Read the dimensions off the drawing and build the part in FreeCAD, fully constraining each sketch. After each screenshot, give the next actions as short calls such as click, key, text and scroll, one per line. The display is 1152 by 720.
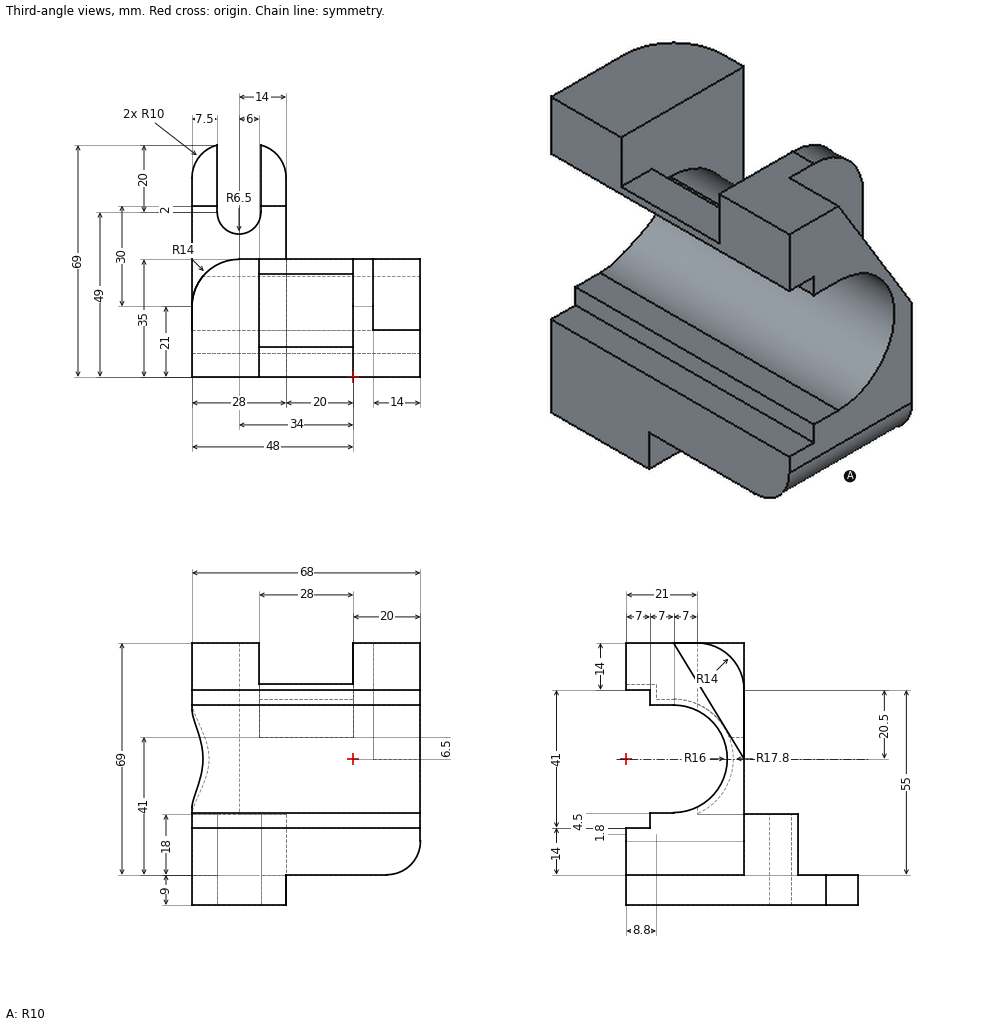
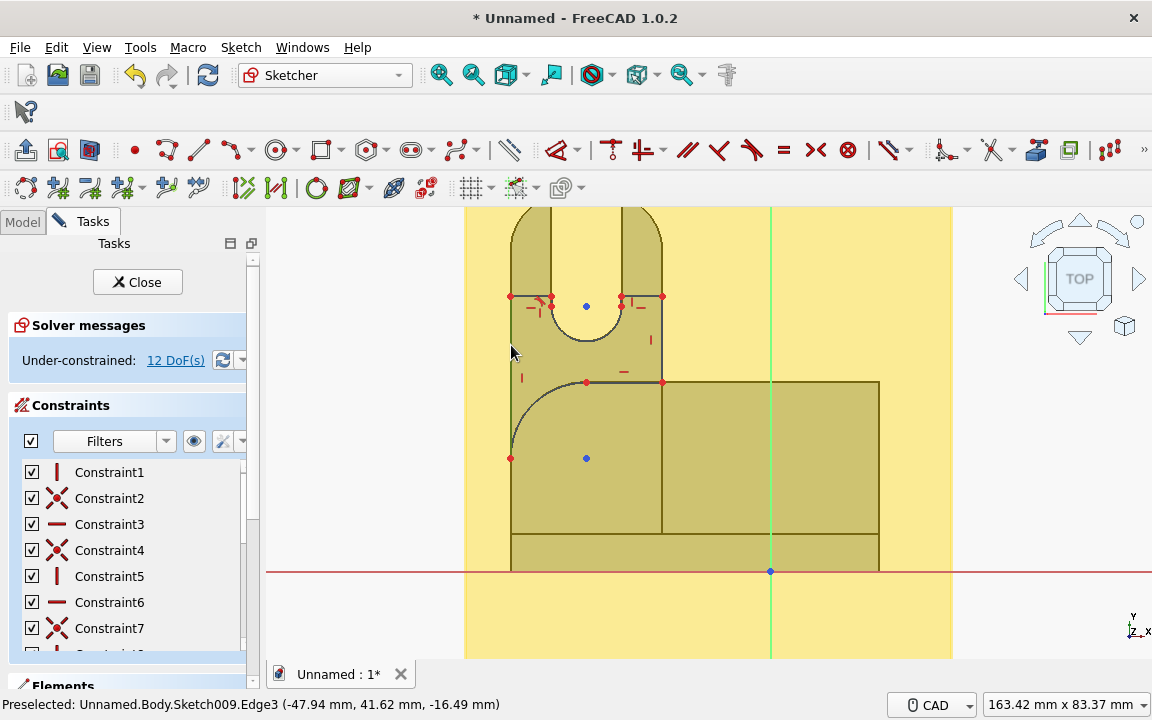
click(552, 391)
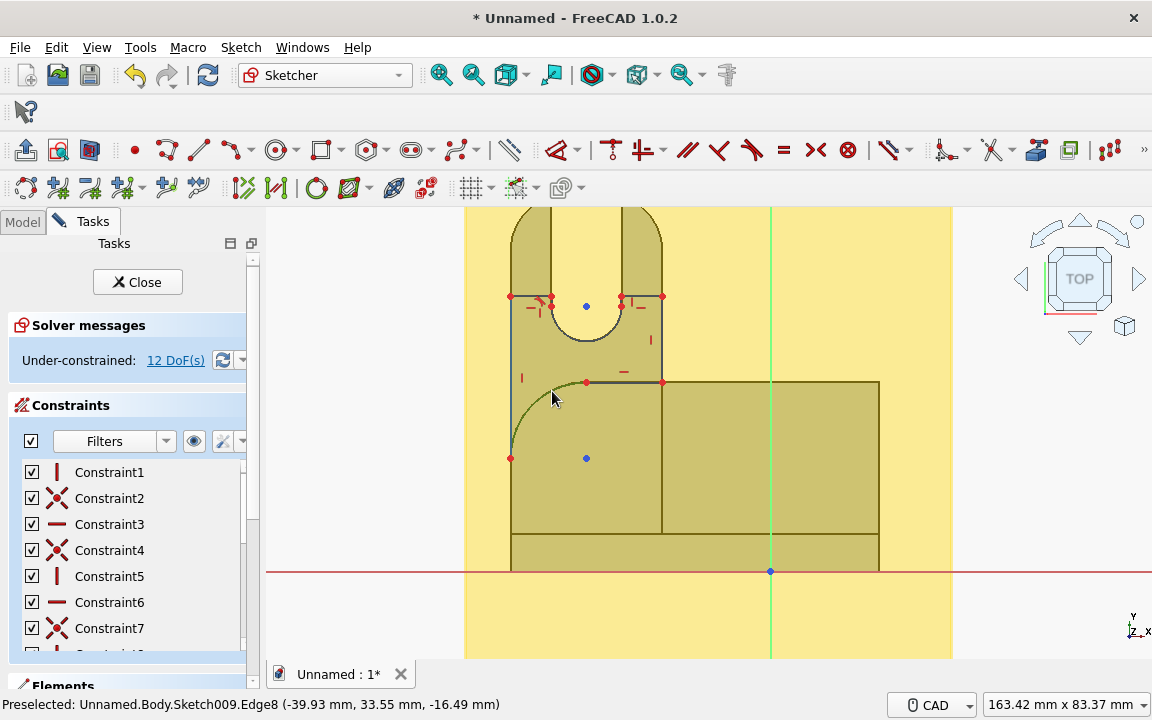
click(752, 150)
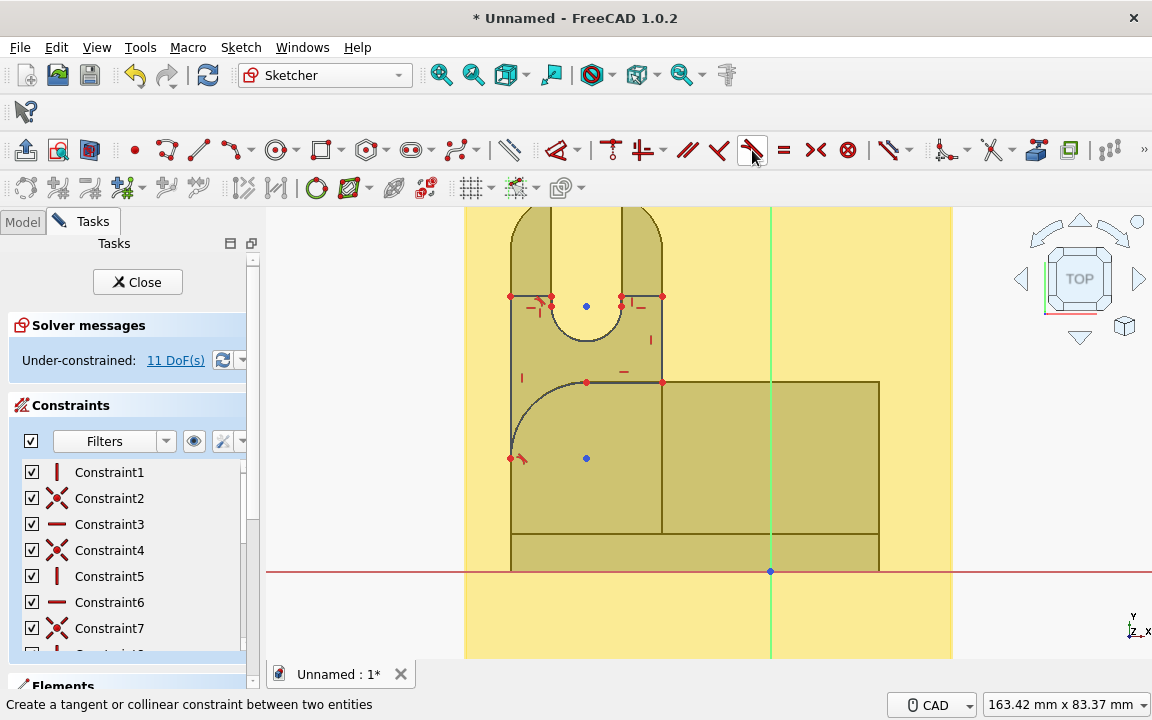
click(609, 383)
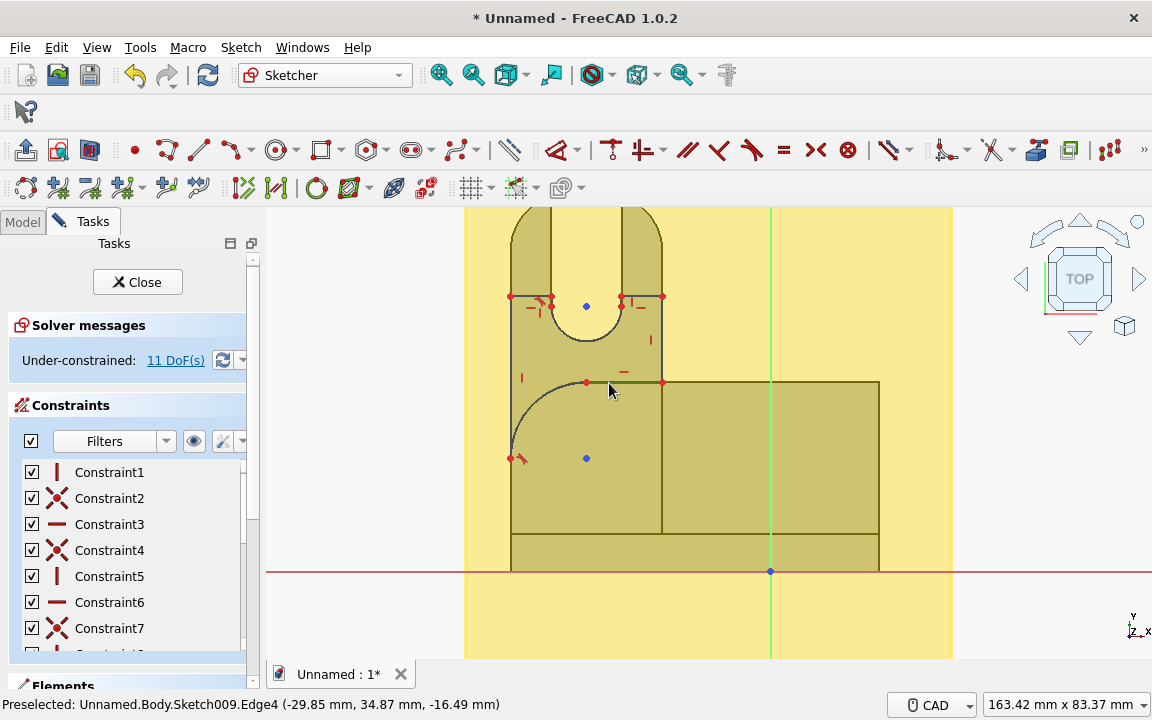
click(552, 391)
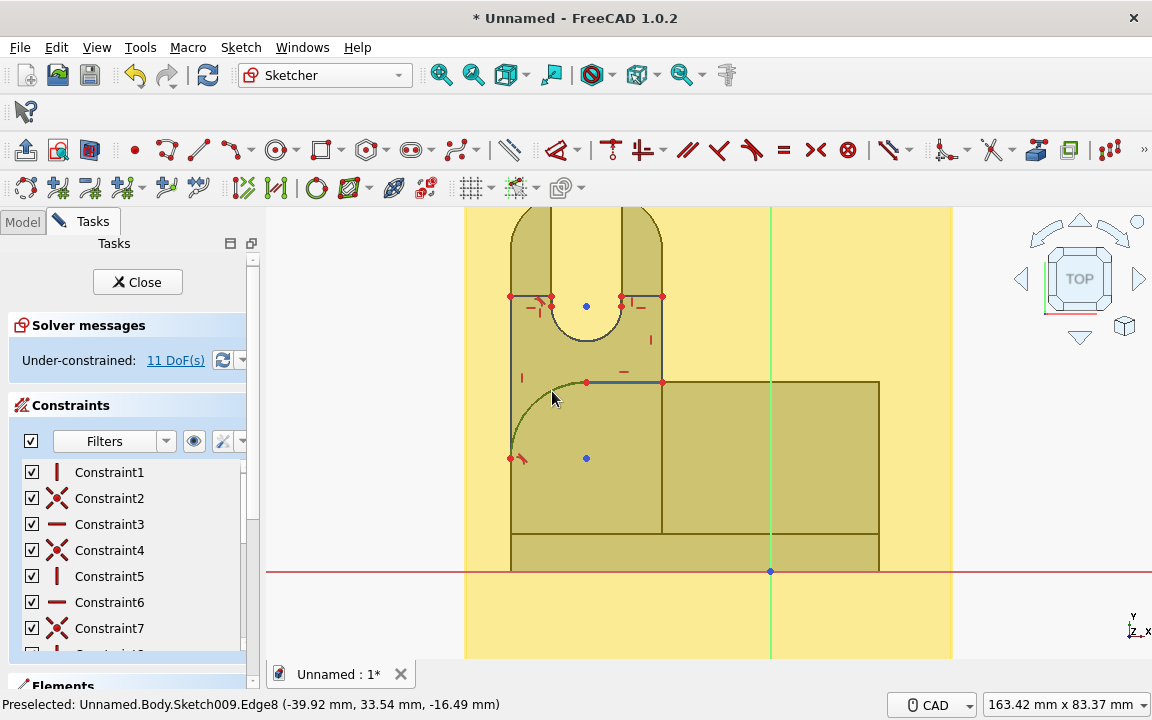
key(t)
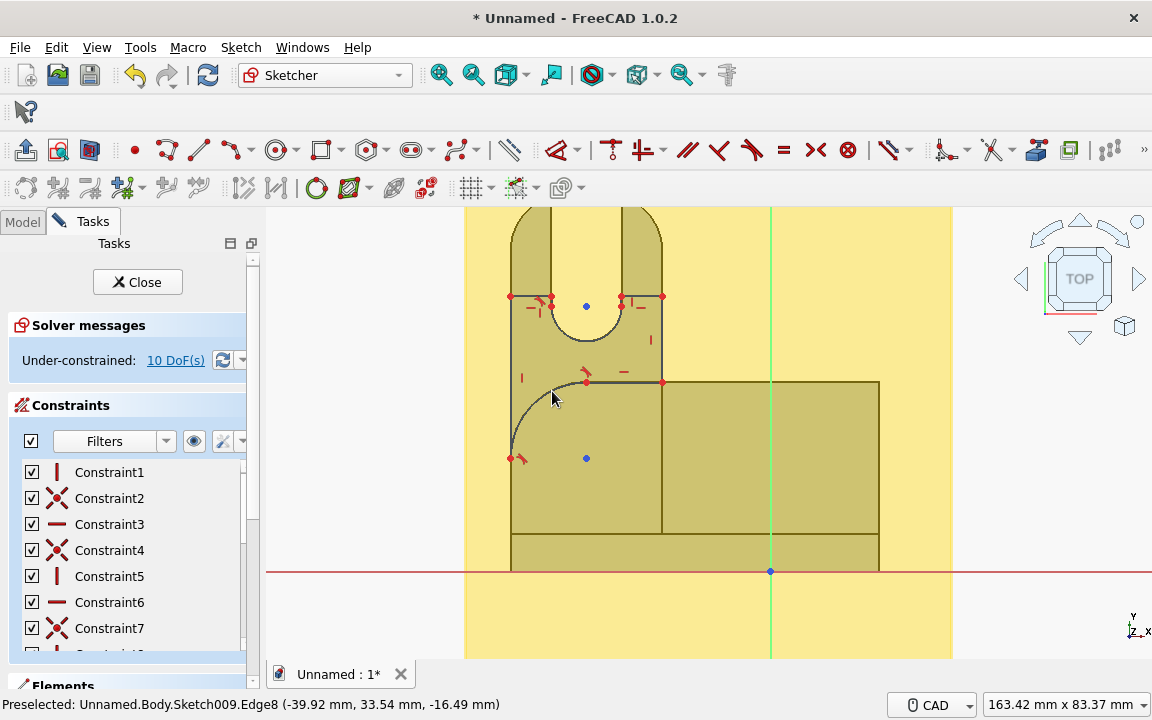
scroll(621, 301, up, 5)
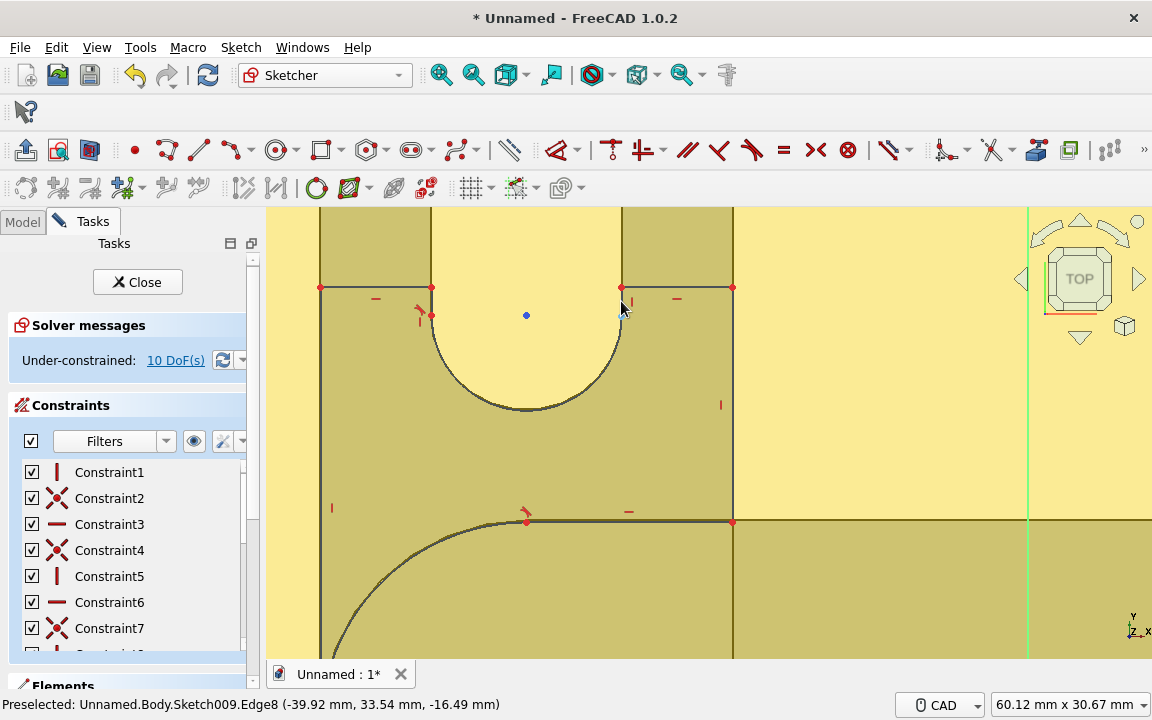
click(622, 302)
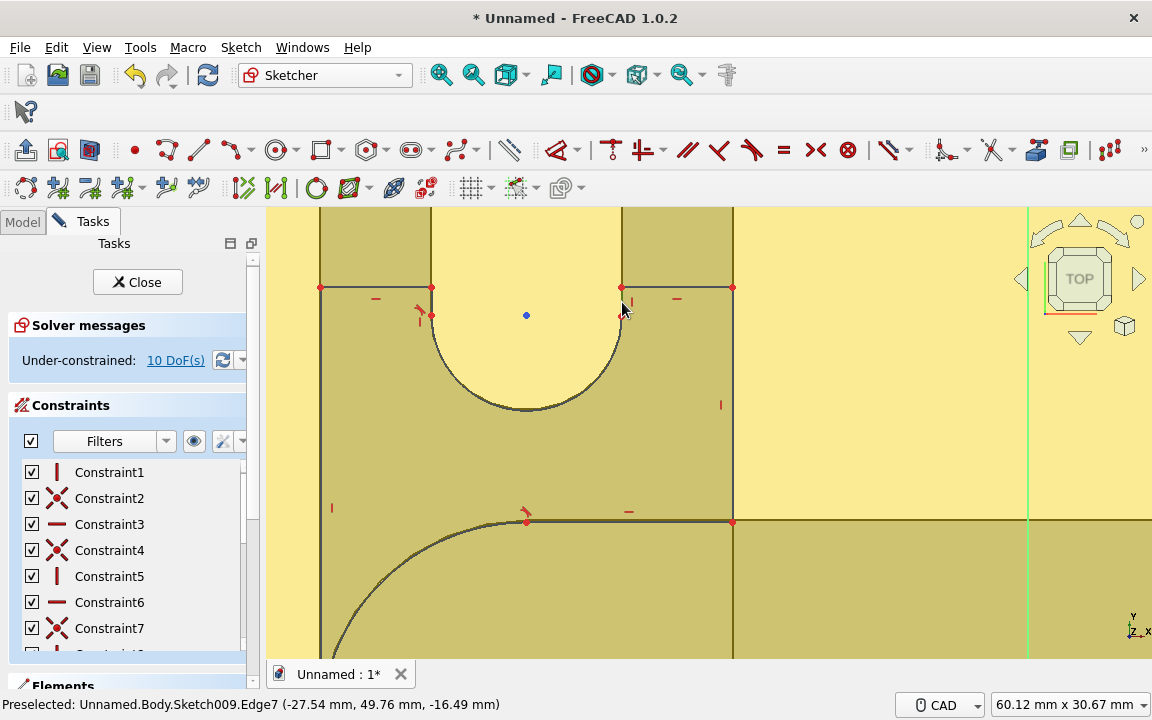
click(471, 392)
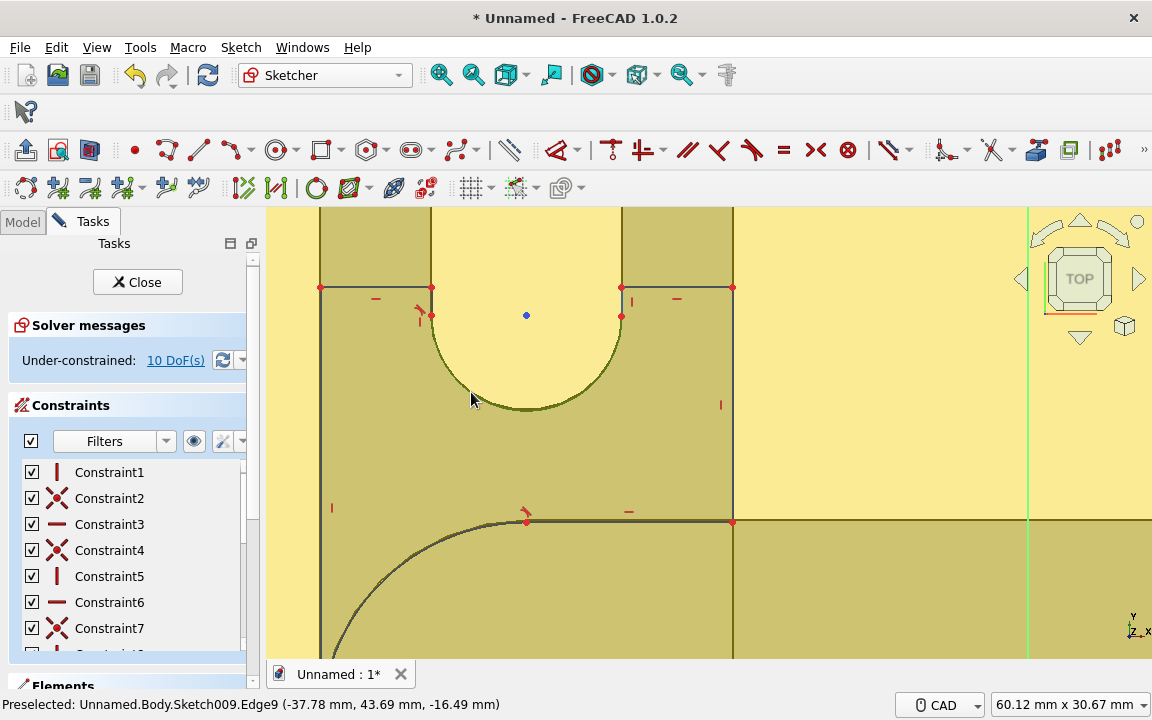
click(752, 150)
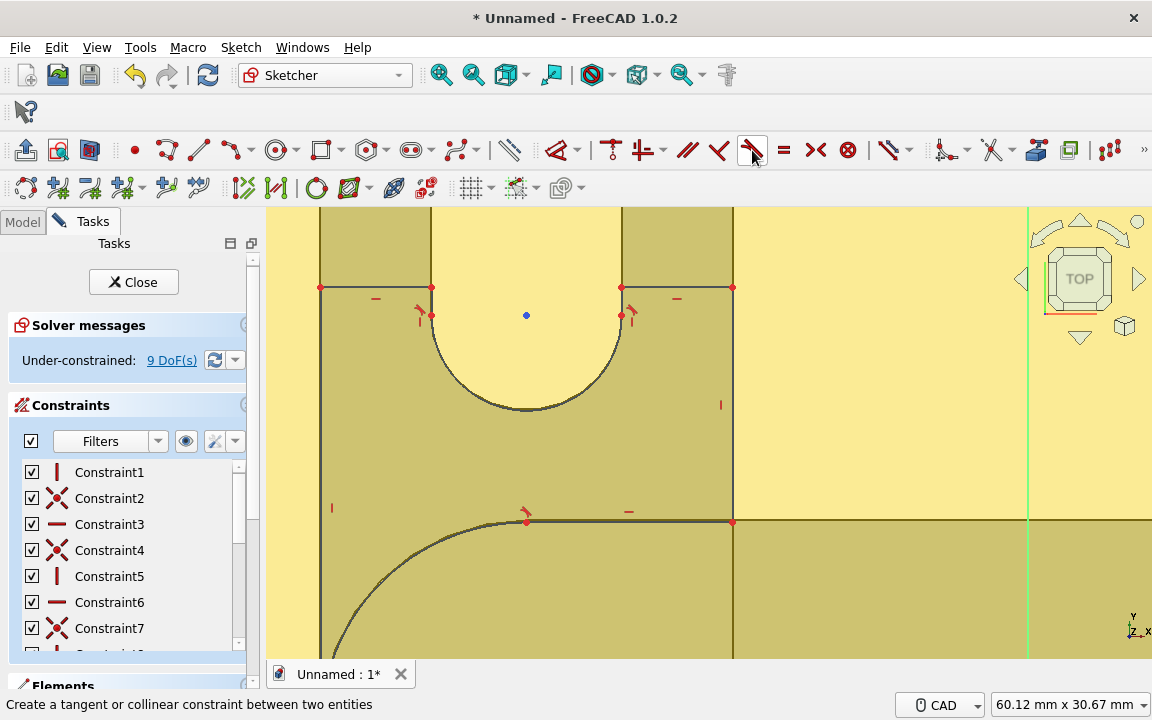
click(556, 150)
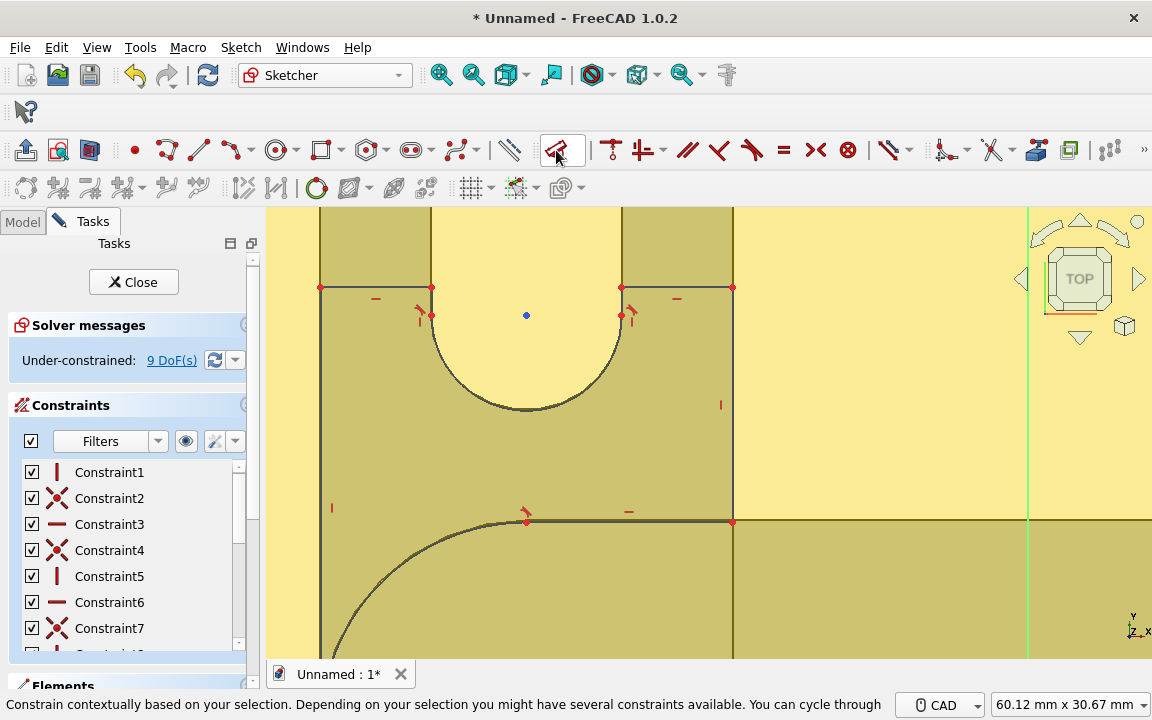
click(433, 545)
click(418, 517)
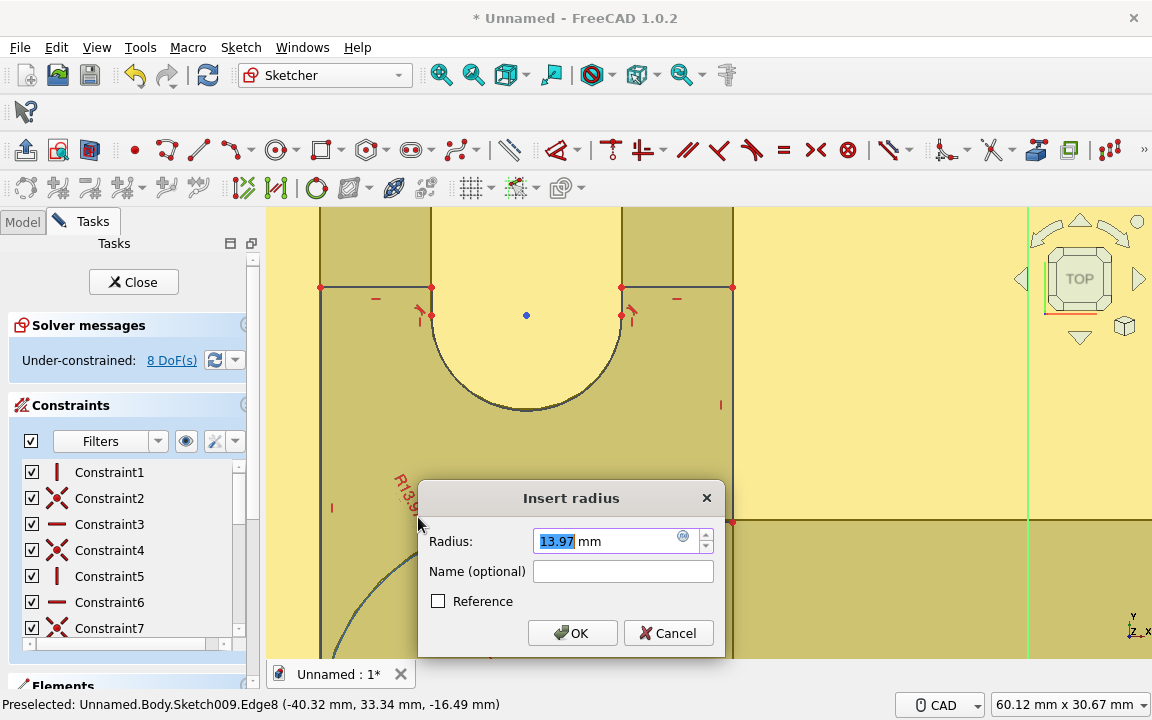
text(14)
key(Return)